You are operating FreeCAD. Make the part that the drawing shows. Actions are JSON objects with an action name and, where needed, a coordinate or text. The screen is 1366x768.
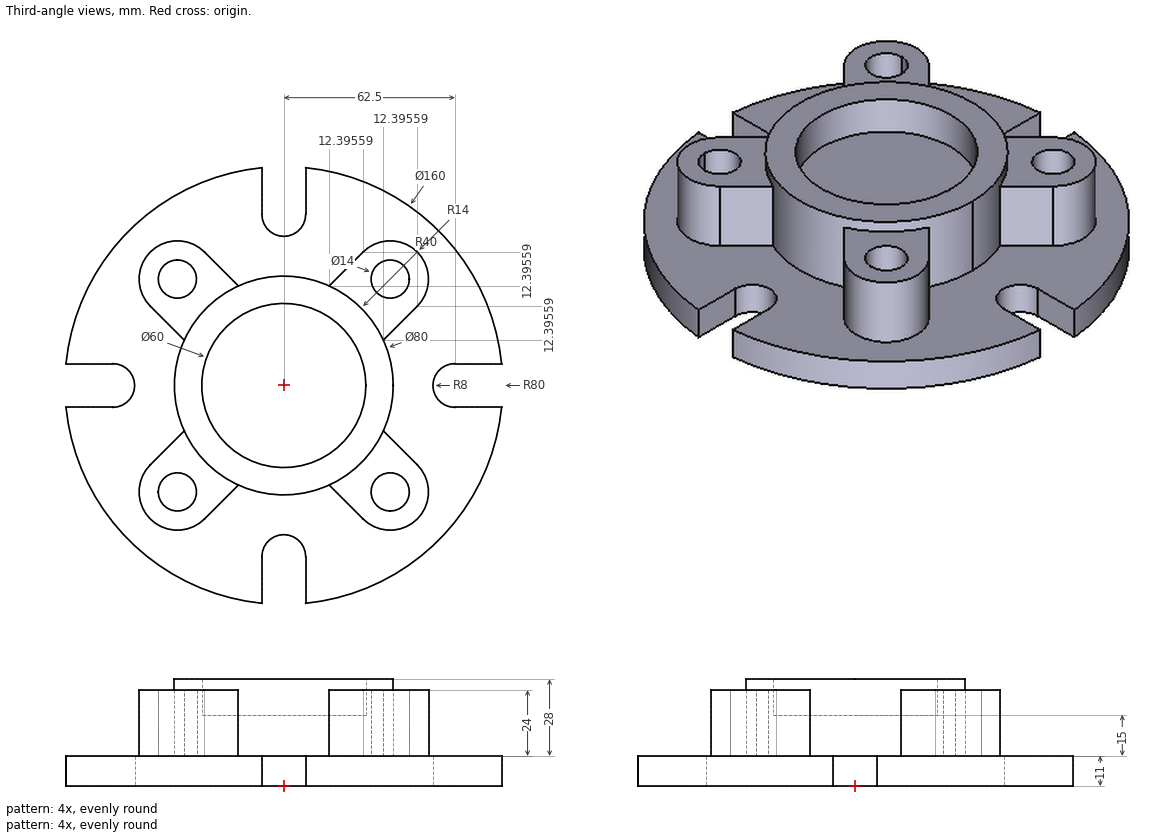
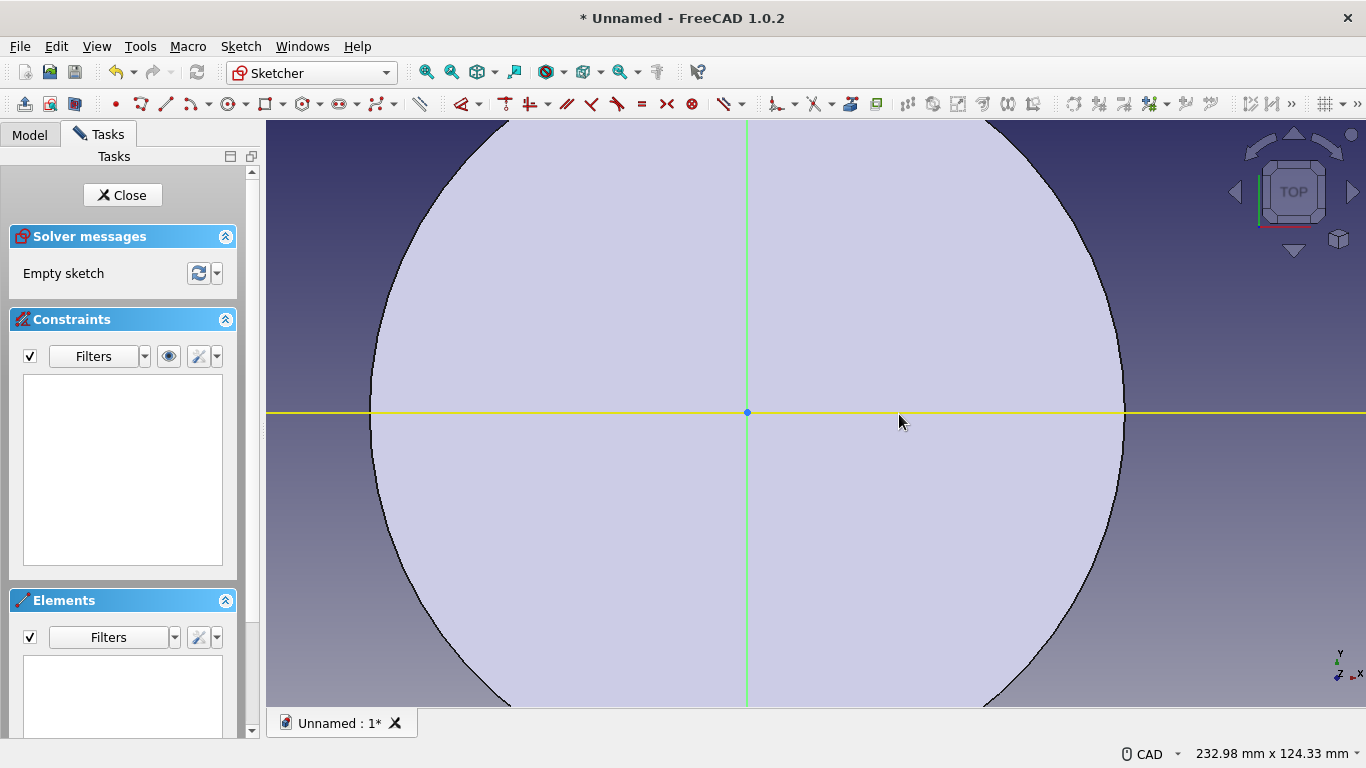
{"action": "key", "text": "g c"}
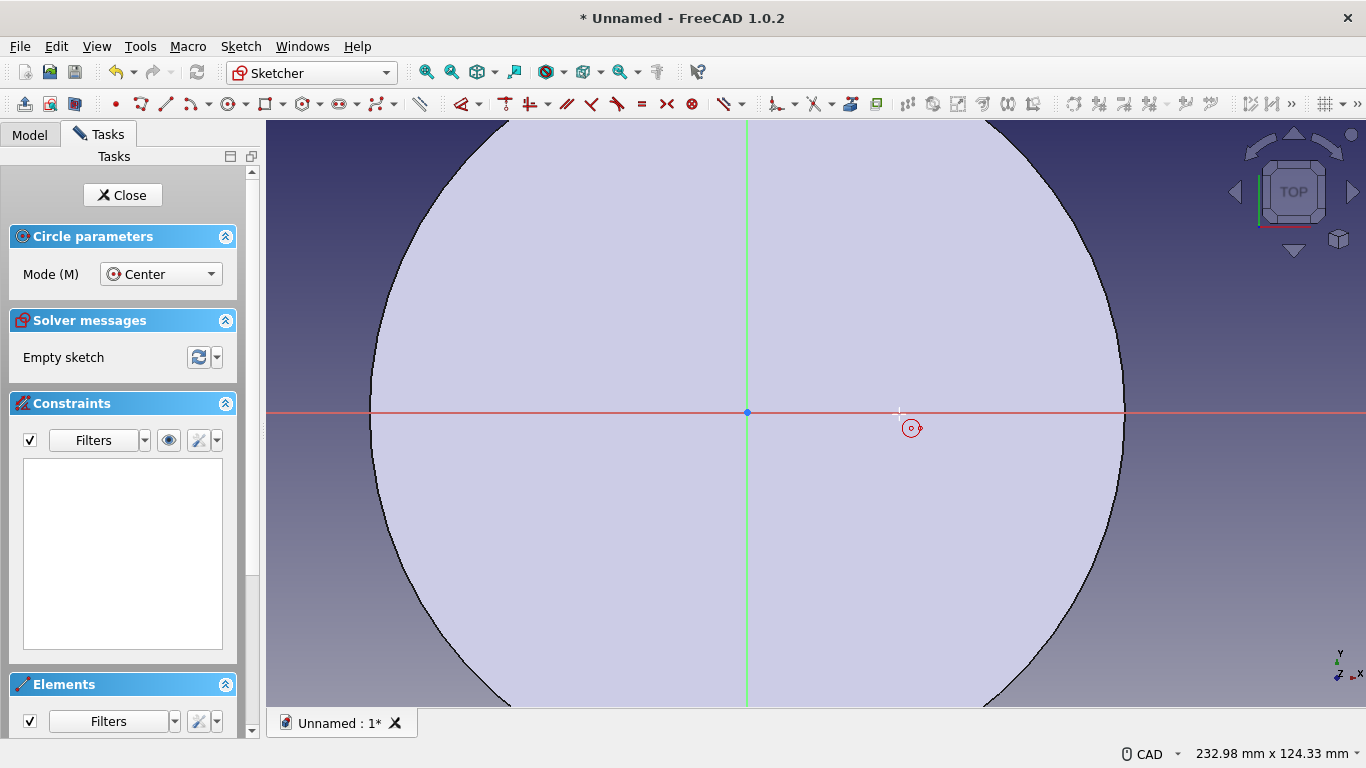
{"action": "left_click", "coordinate": [747, 413]}
{"action": "left_click", "coordinate": [881, 279]}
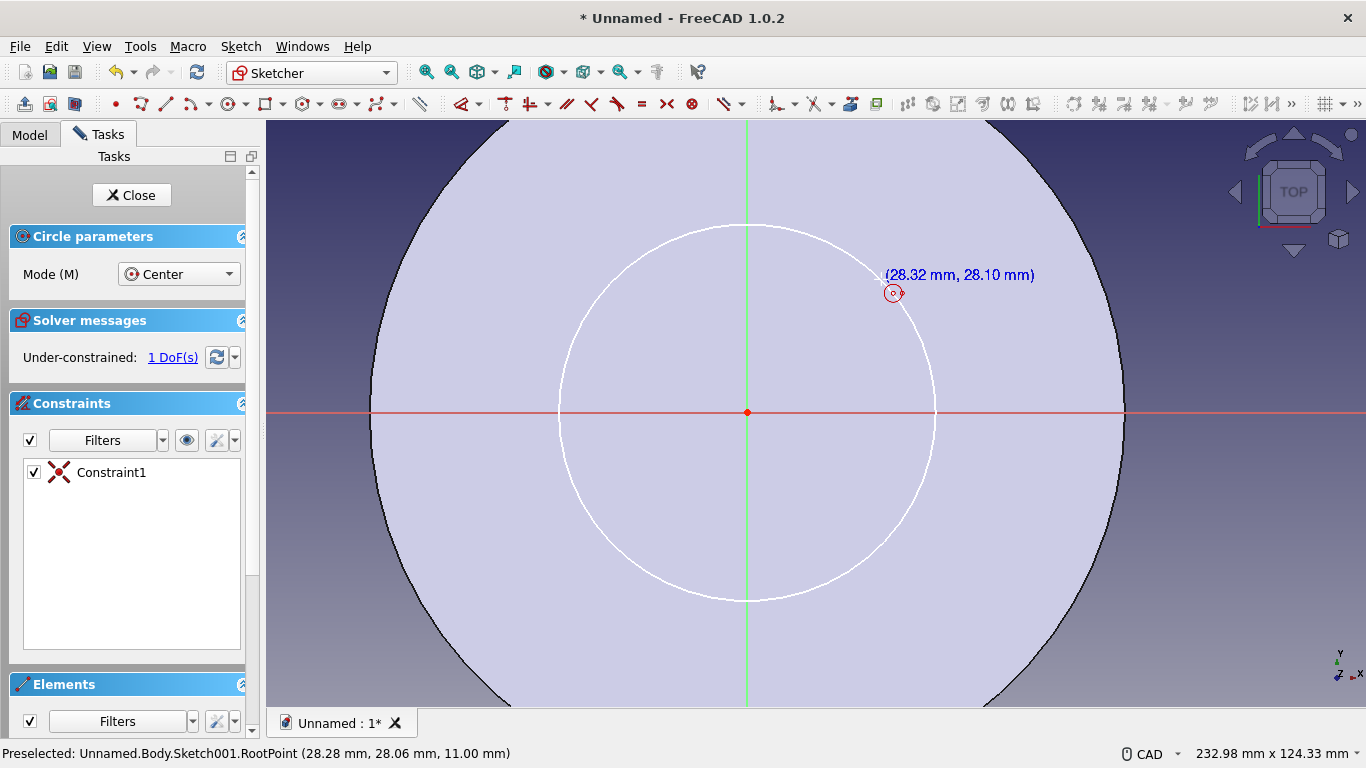
{"action": "left_click", "coordinate": [747, 413]}
{"action": "left_click", "coordinate": [847, 313]}
{"action": "key", "text": "Escape"}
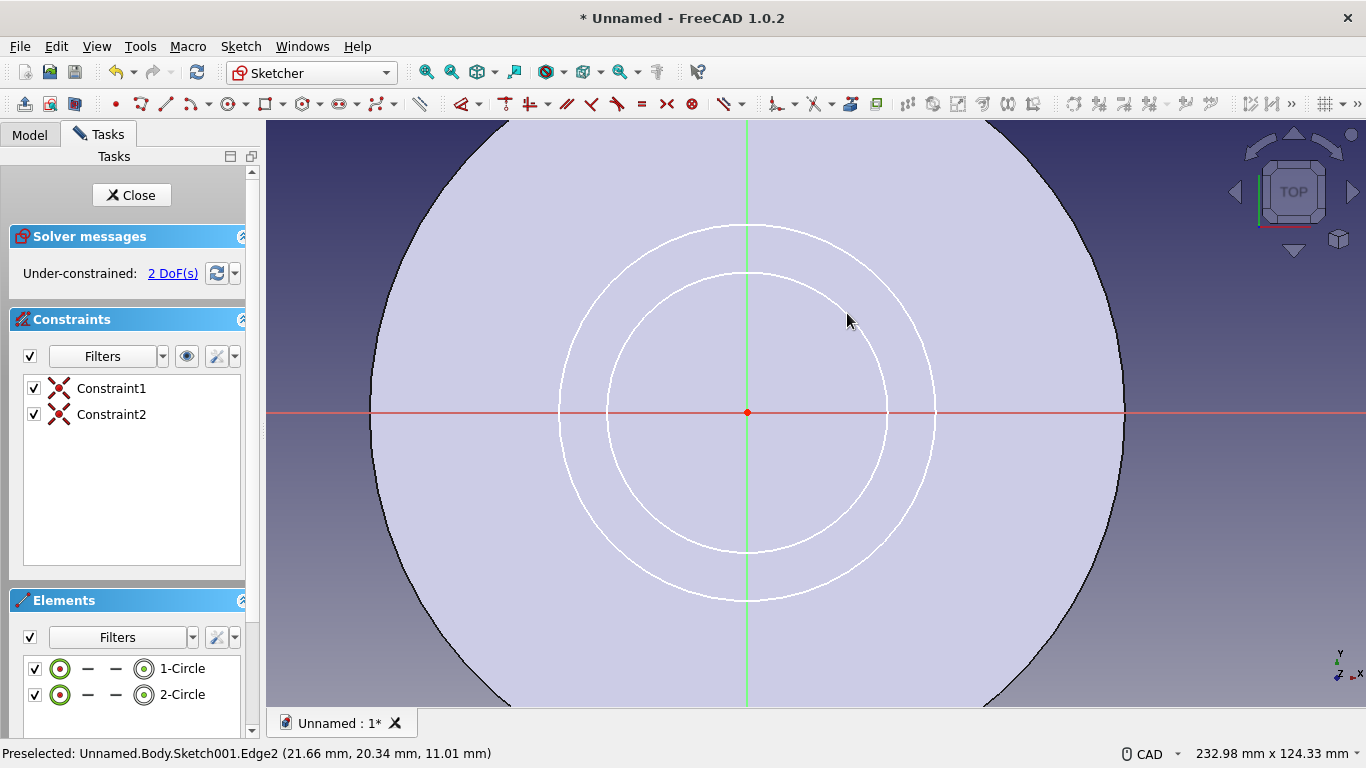
{"action": "key", "text": "d"}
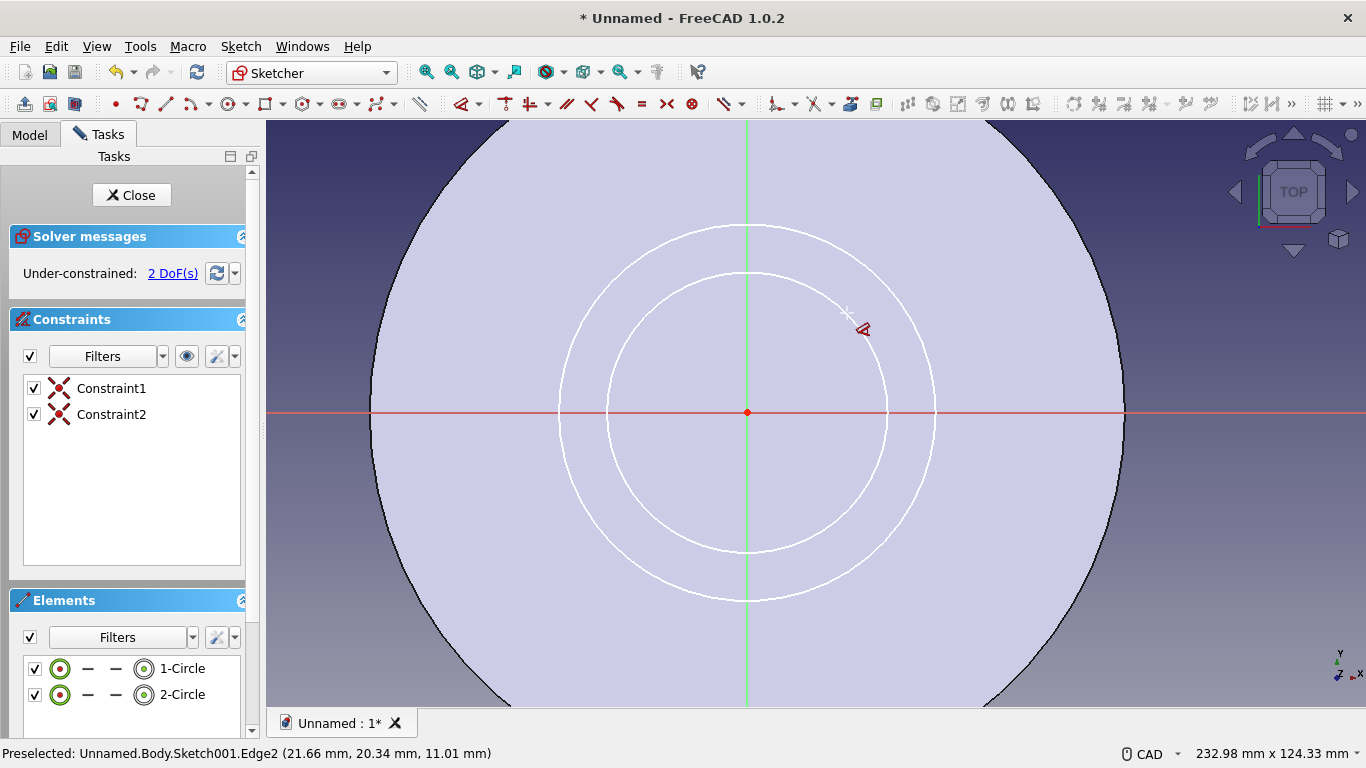
{"action": "left_click", "coordinate": [880, 279]}
{"action": "left_click", "coordinate": [903, 256]}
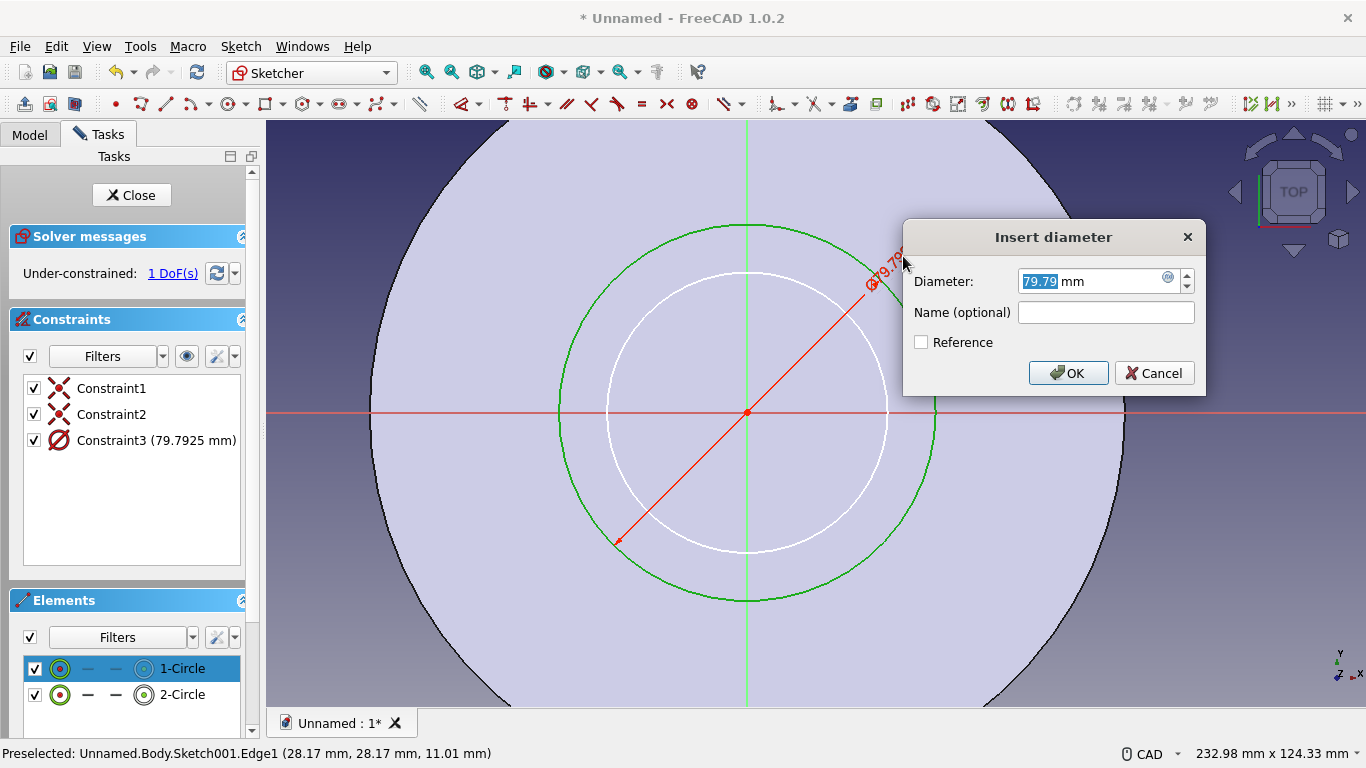
{"action": "type", "text": "80"}
{"action": "key", "text": "Return"}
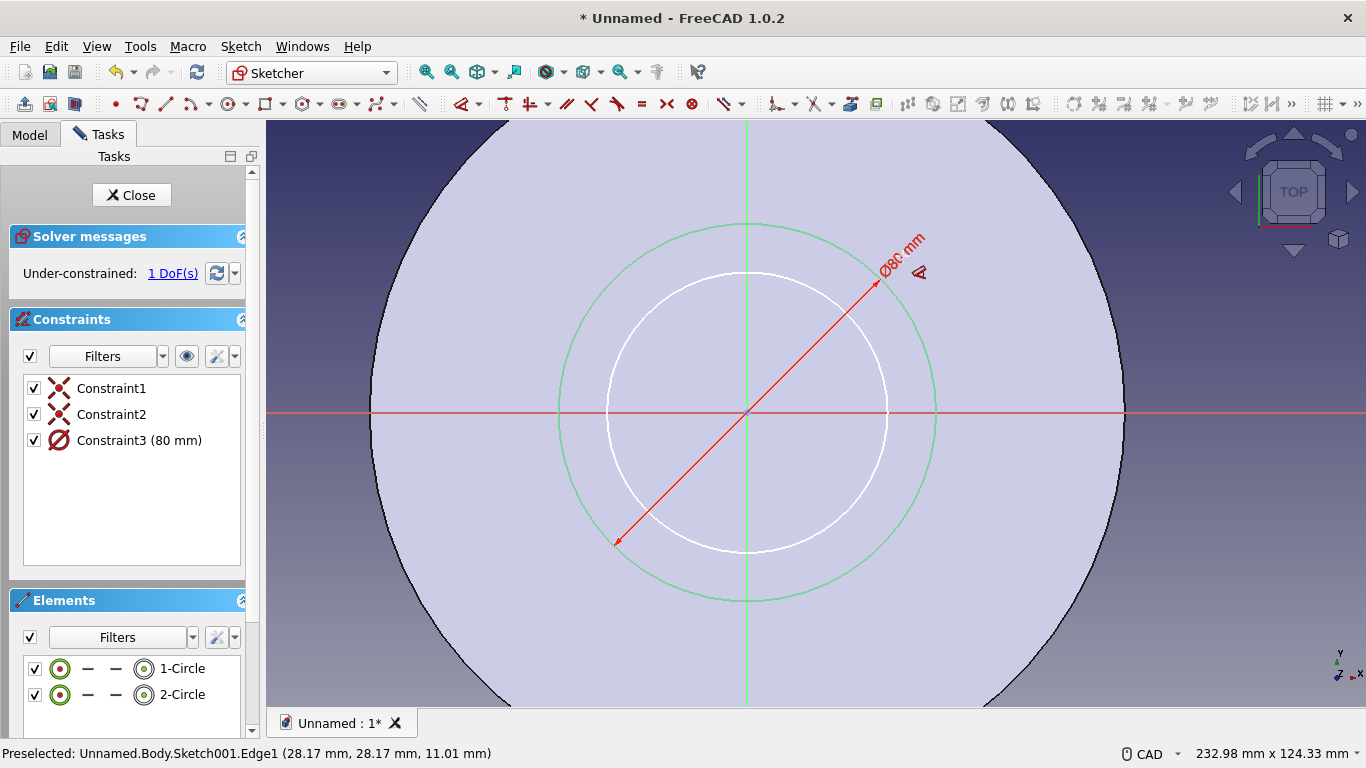
{"action": "left_click", "coordinate": [846, 313]}
{"action": "left_click", "coordinate": [869, 290]}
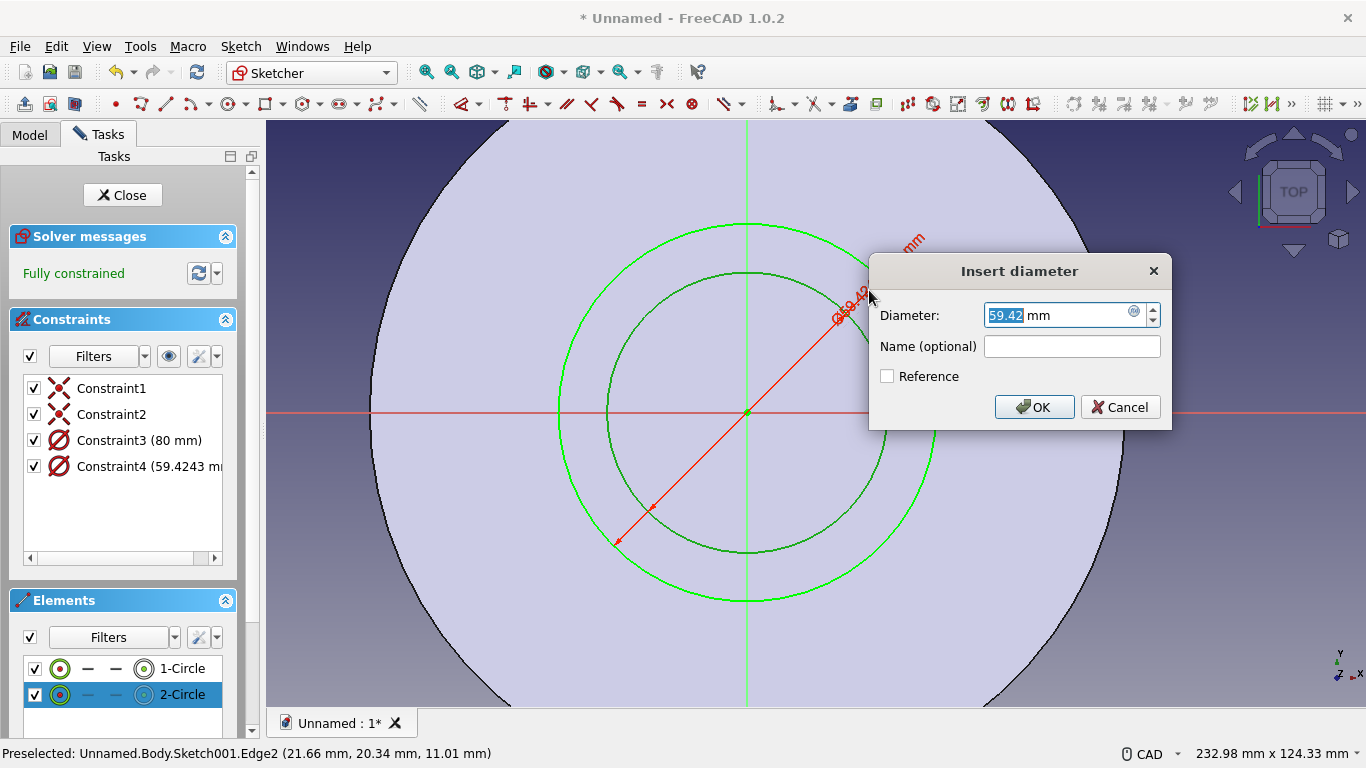
{"action": "type", "text": "60"}
{"action": "key", "text": "Return"}
{"action": "key", "text": "Escape"}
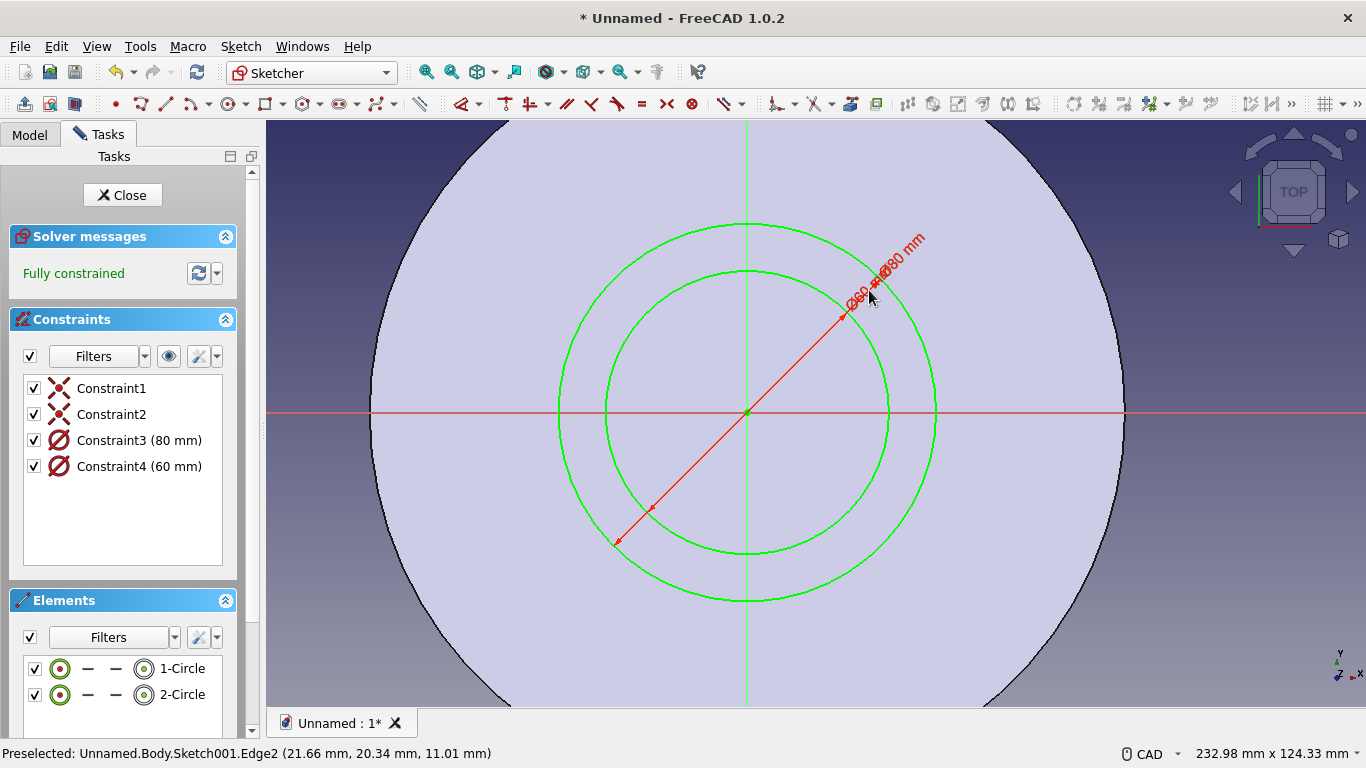
{"action": "left_click", "coordinate": [123, 195]}